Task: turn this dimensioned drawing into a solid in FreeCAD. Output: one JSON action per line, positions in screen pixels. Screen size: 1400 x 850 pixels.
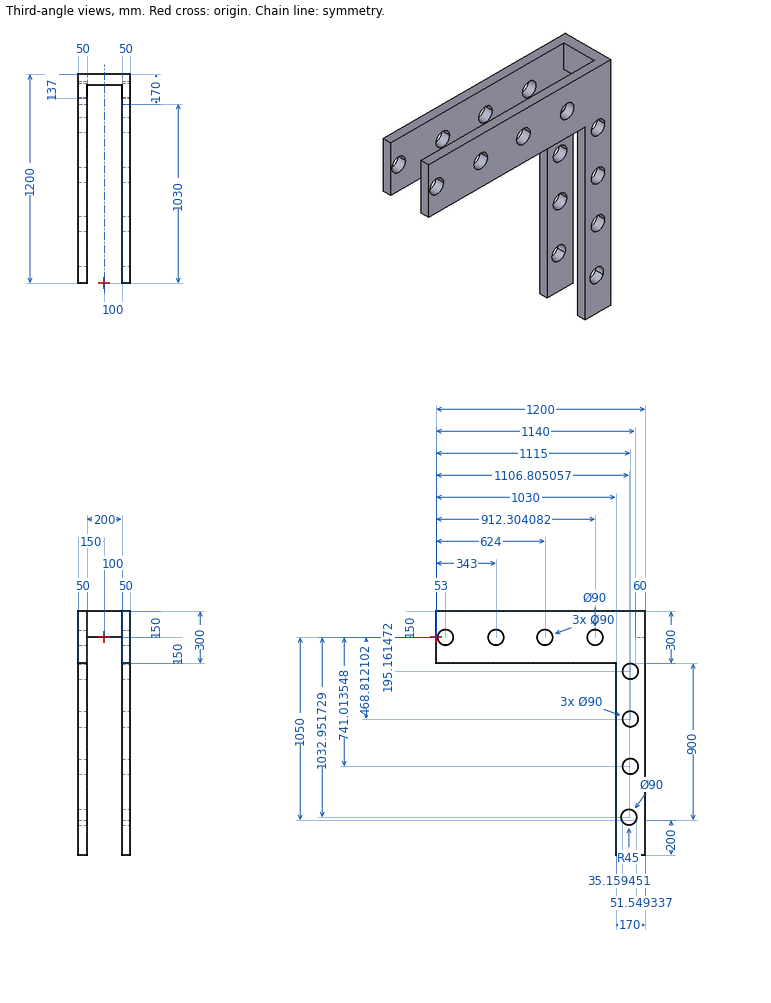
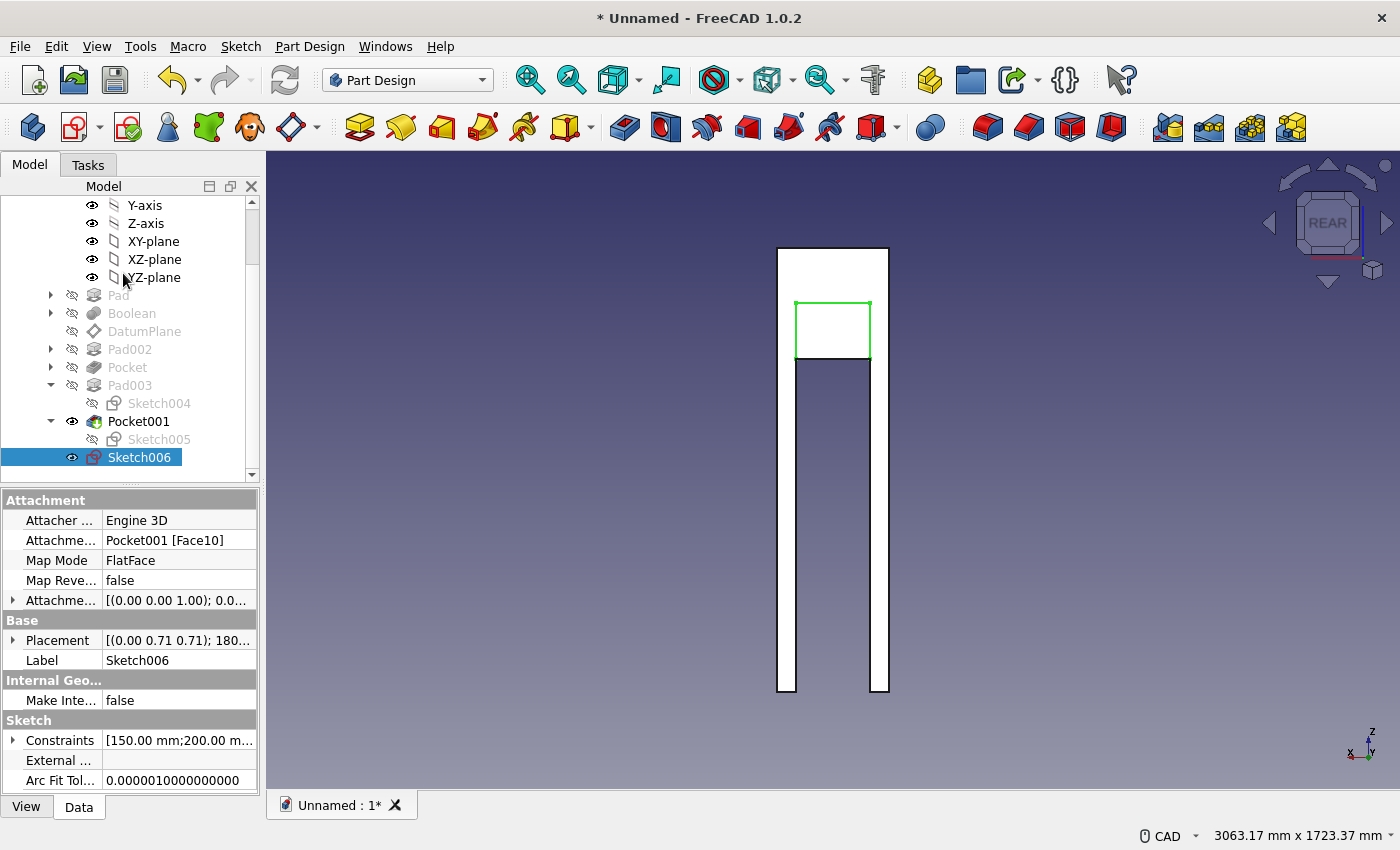
{"action": "left_click", "coordinate": [625, 128]}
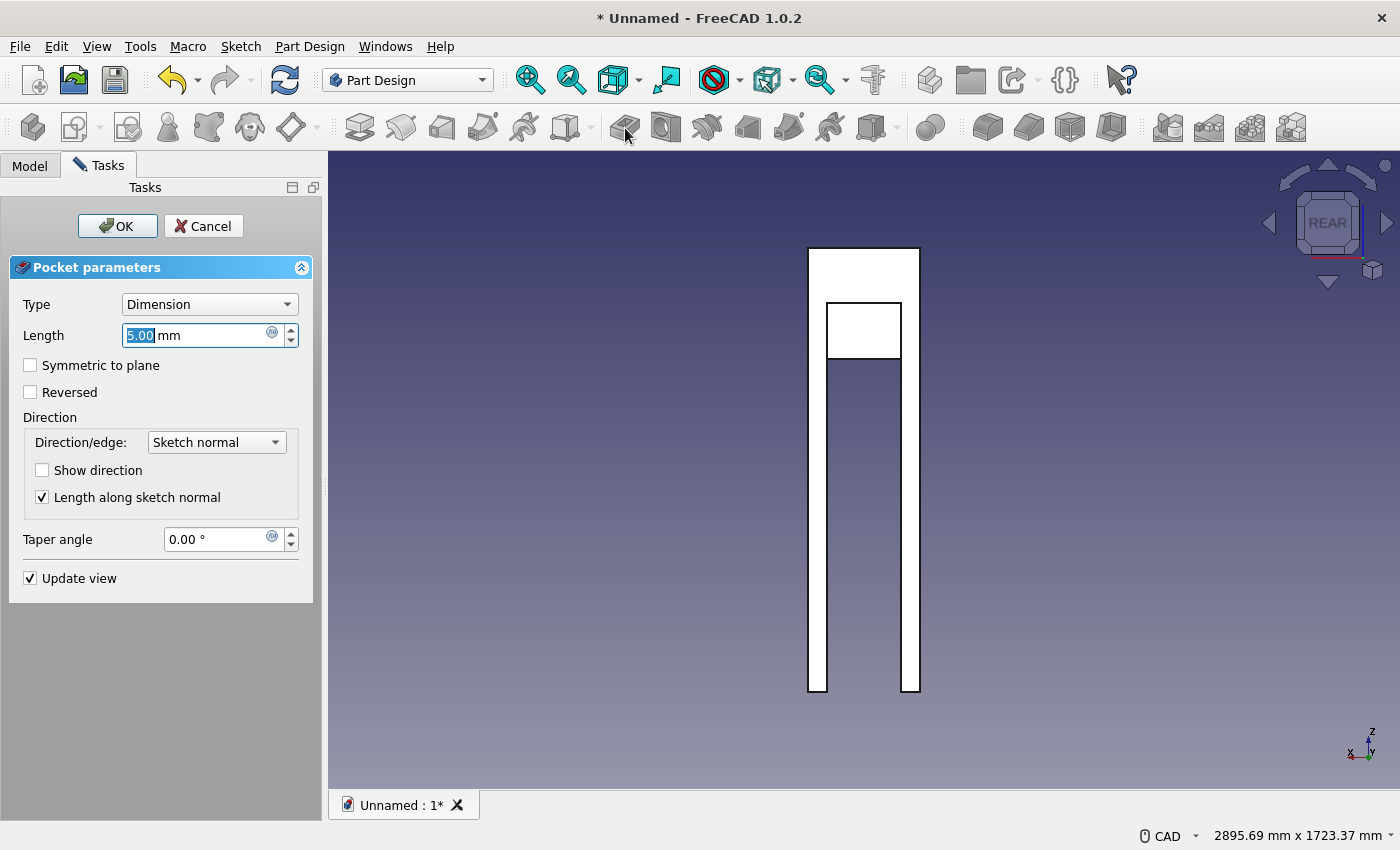
{"action": "type", "text": "137"}
{"action": "key", "text": "Tab"}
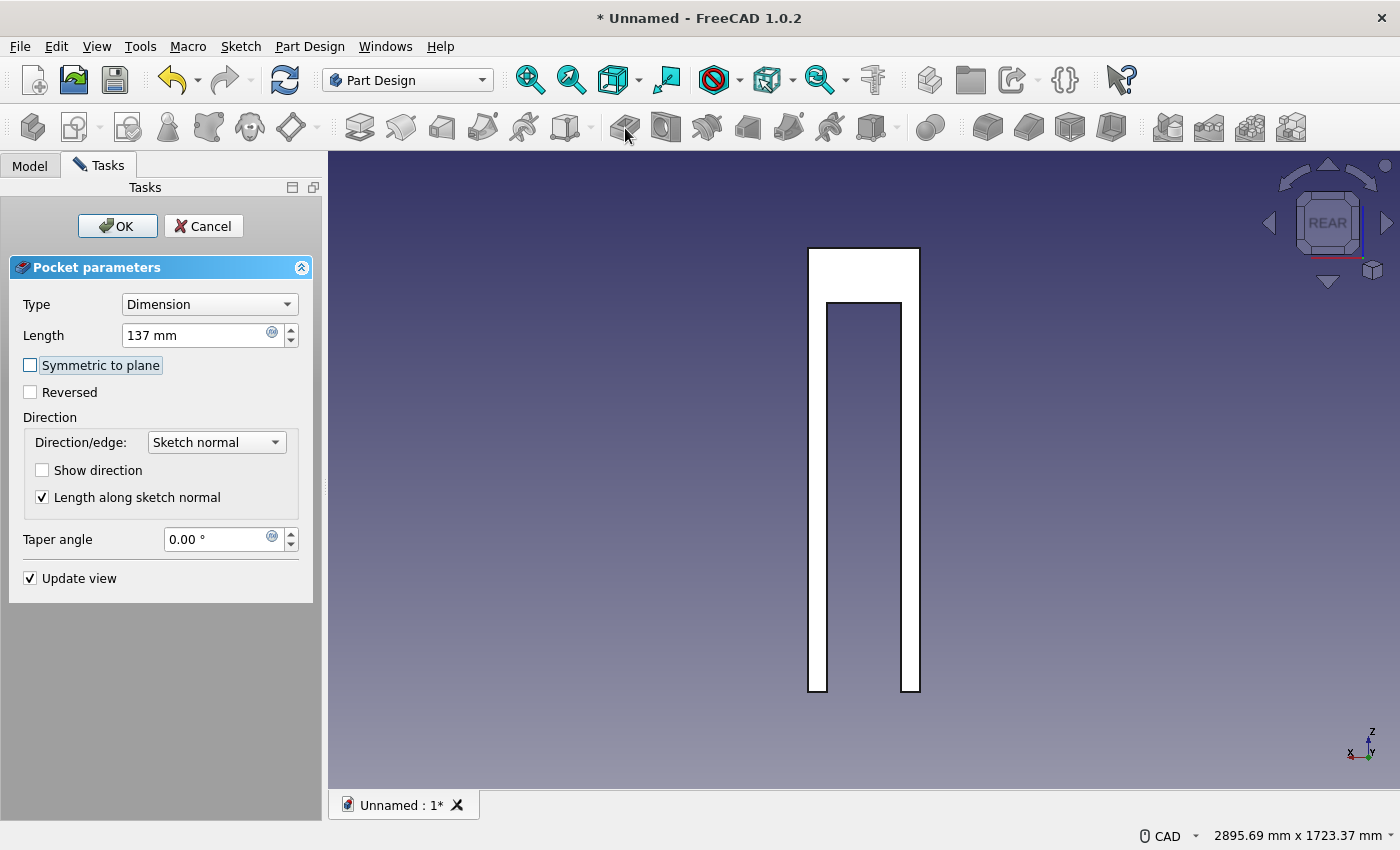
{"action": "left_click", "coordinate": [118, 226]}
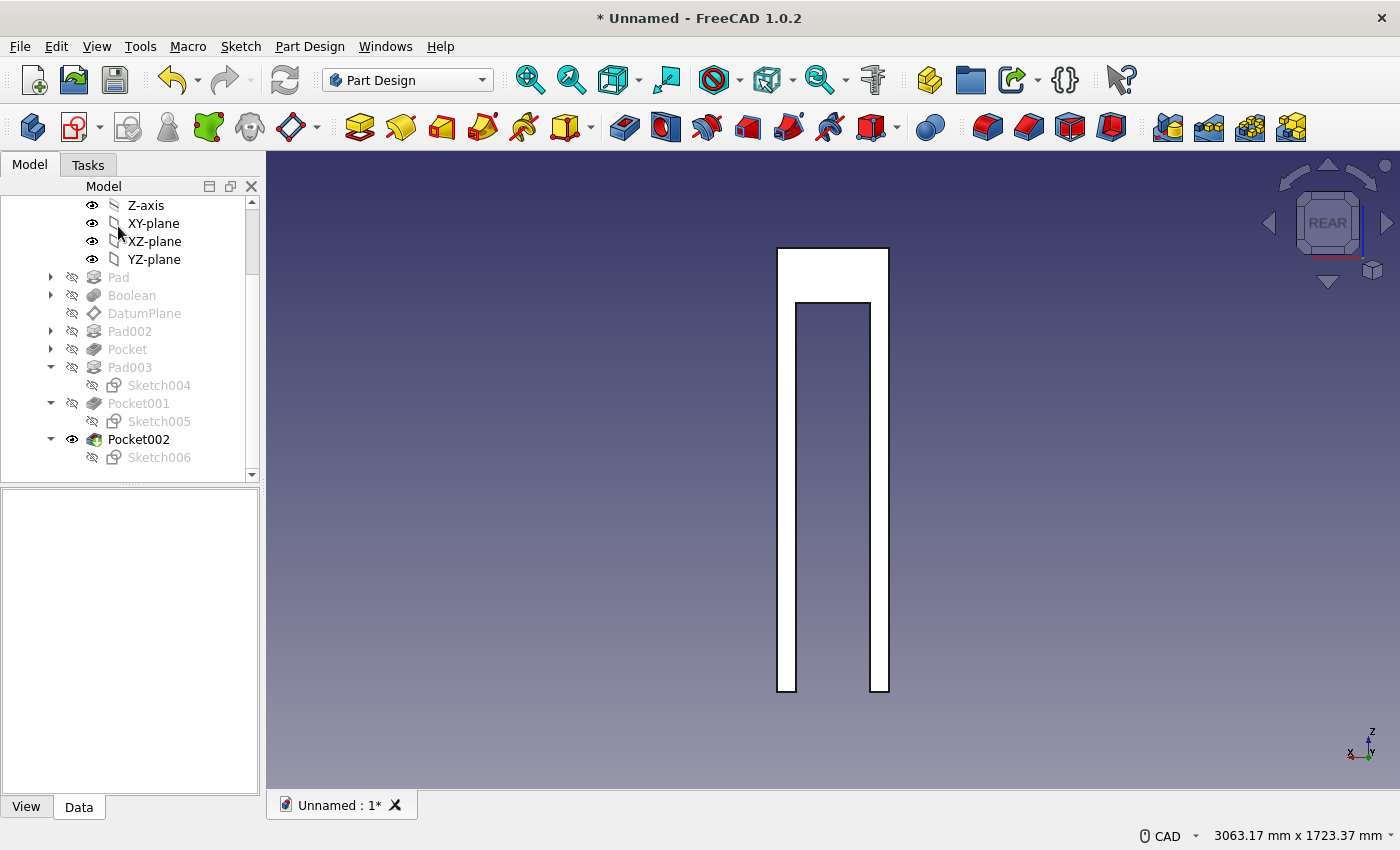
{"action": "key", "text": "0"}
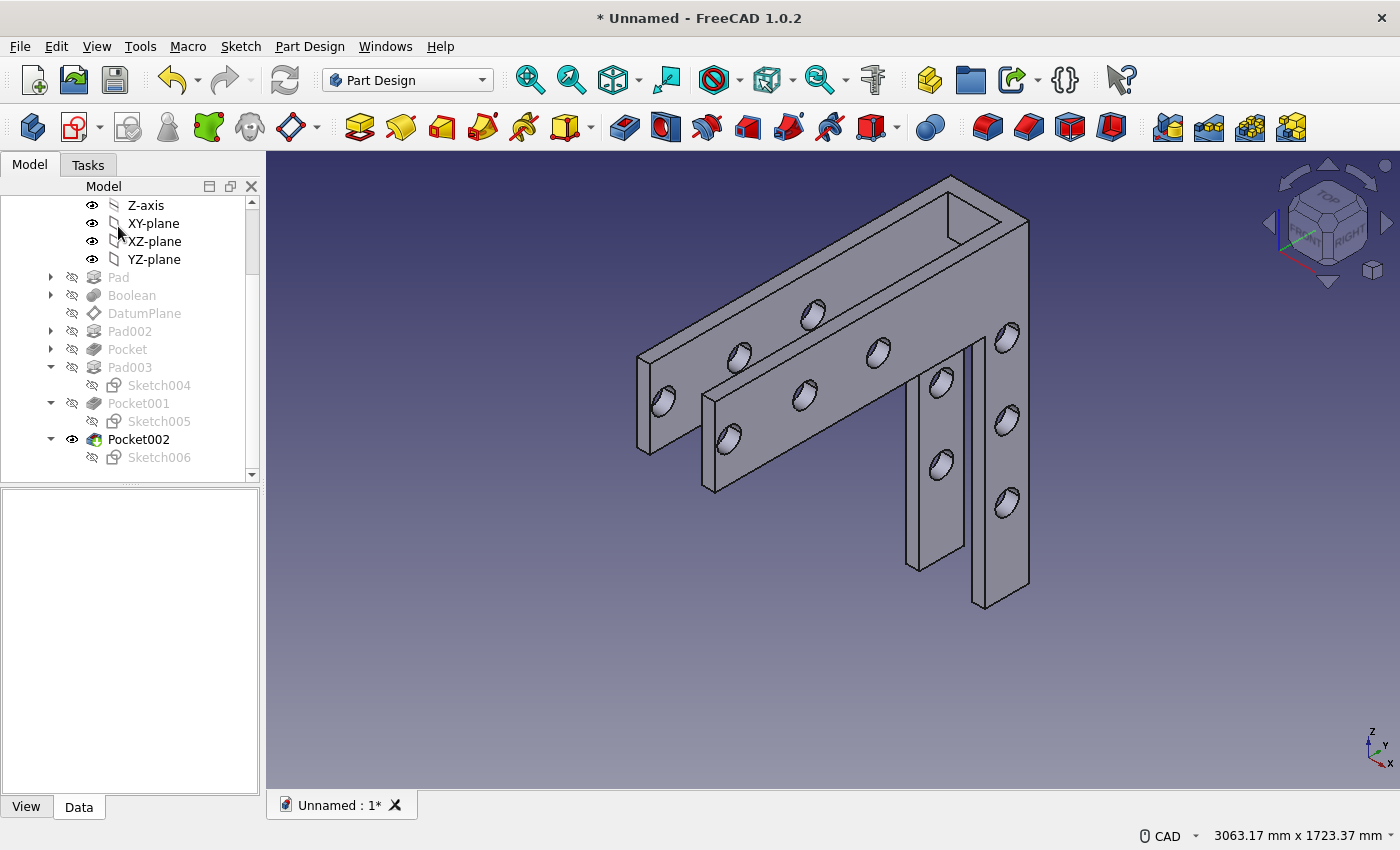
{"action": "left_click", "coordinate": [917, 310]}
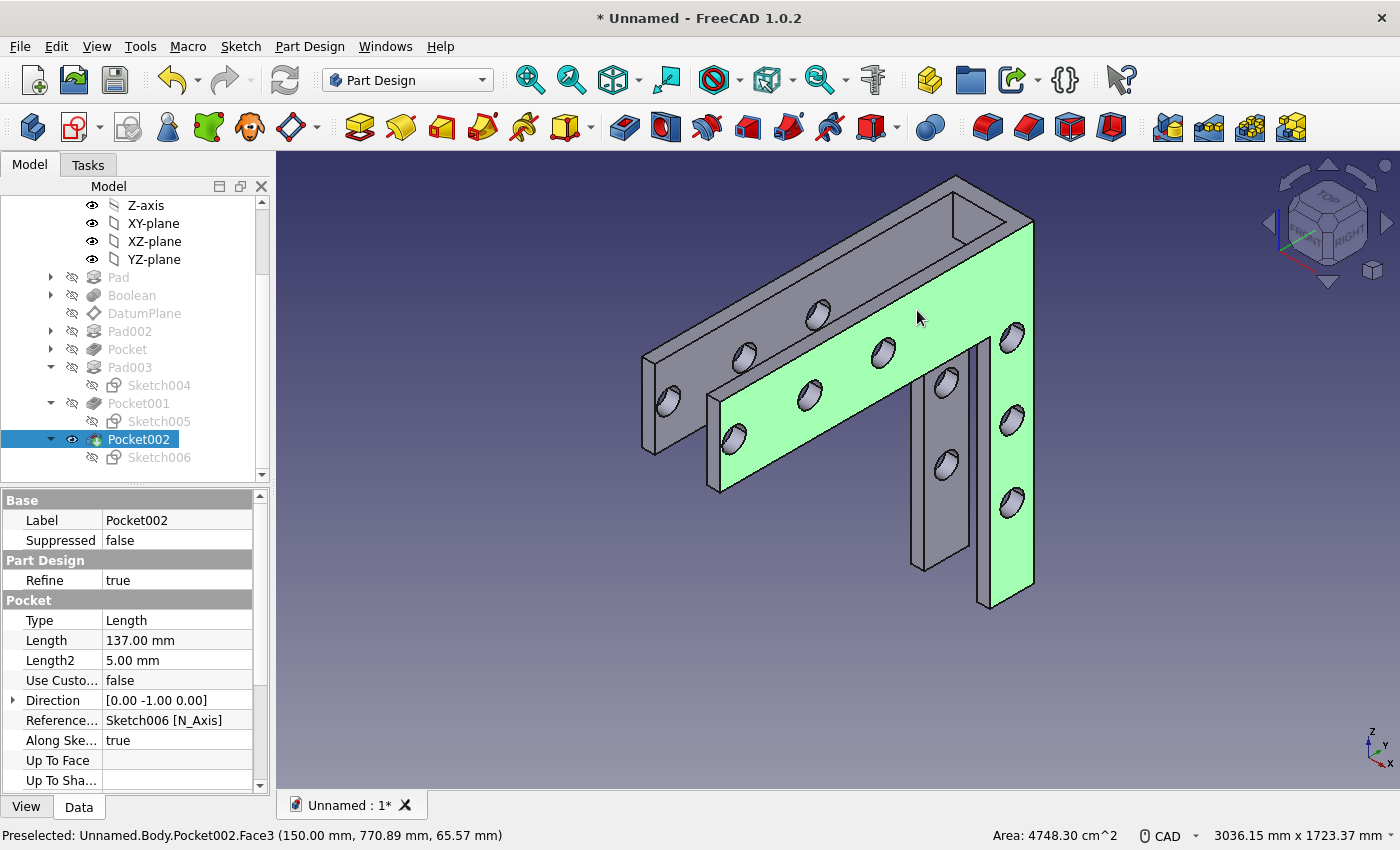
{"action": "left_click", "coordinate": [74, 128]}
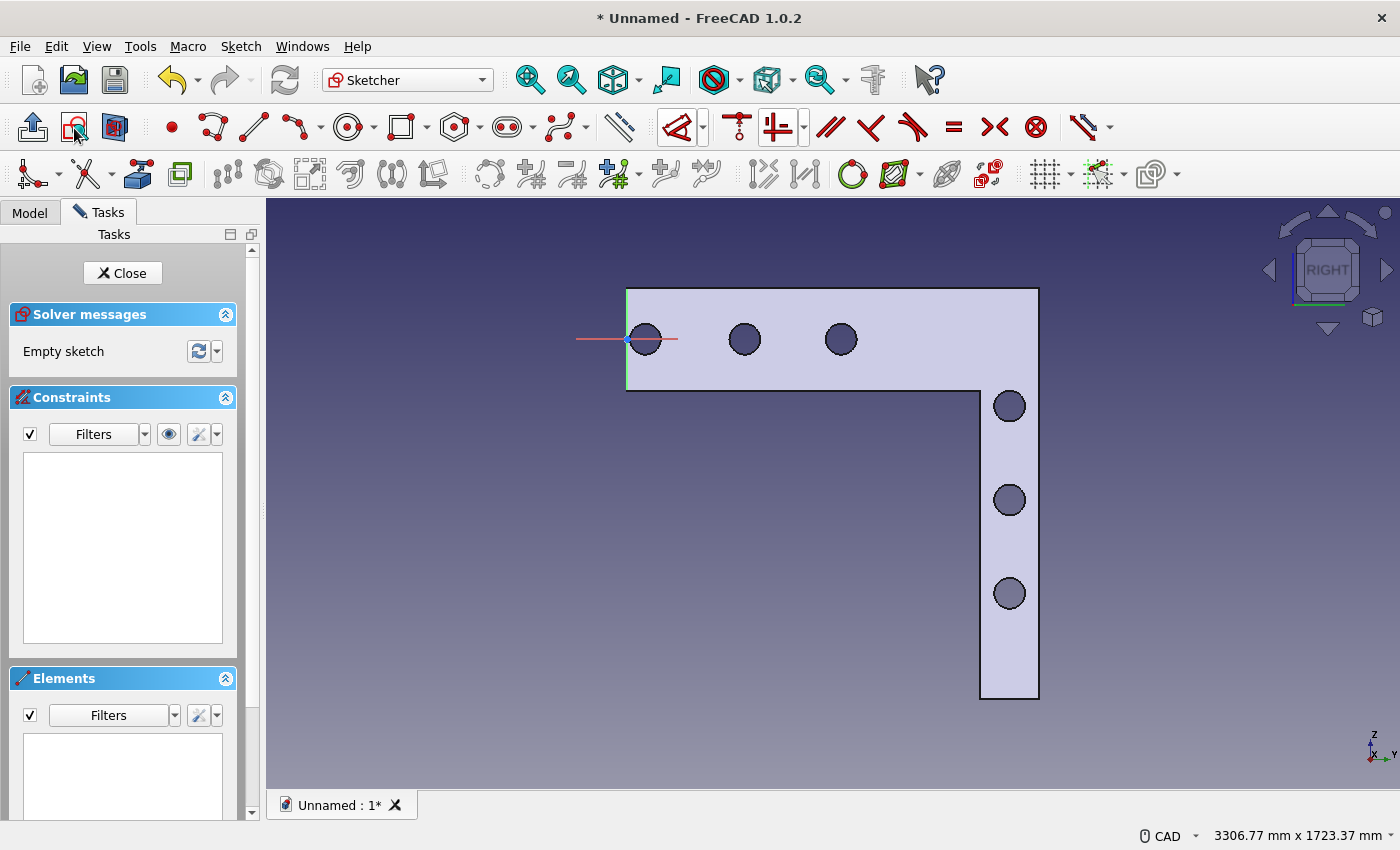
{"action": "scroll", "coordinate": [1026, 709], "scroll_direction": "up", "scroll_amount": 13}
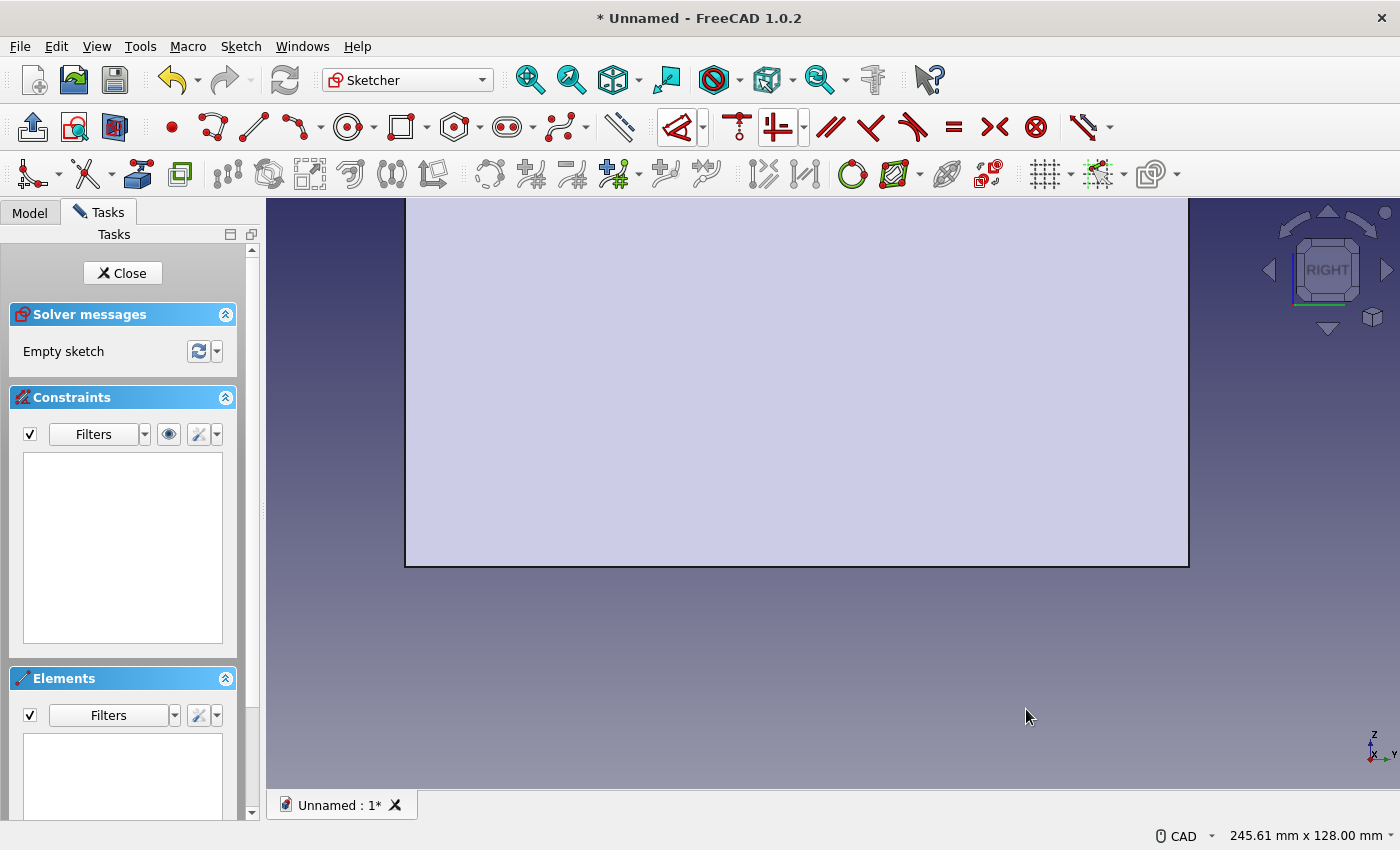
{"action": "left_click", "coordinate": [348, 128]}